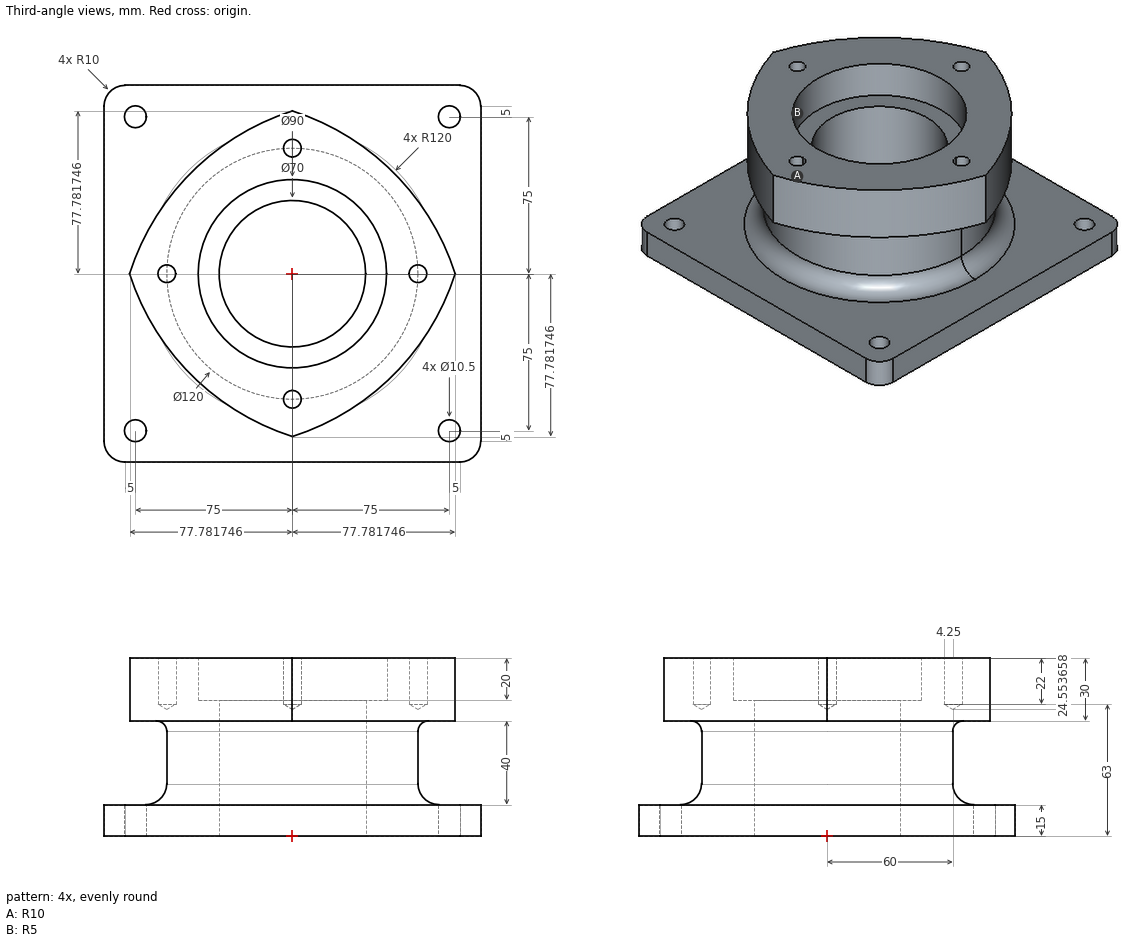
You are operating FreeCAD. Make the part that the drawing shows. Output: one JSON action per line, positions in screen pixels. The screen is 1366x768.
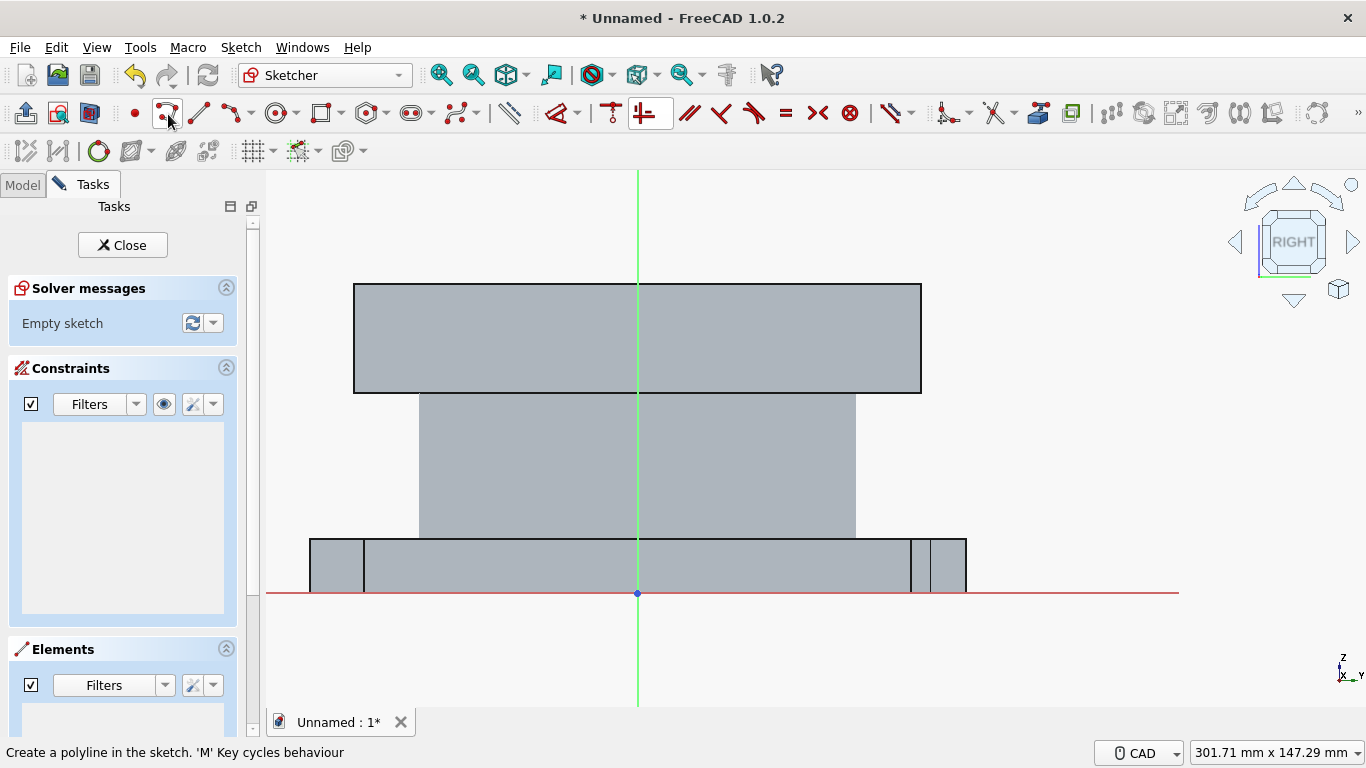
{"action": "left_click", "coordinate": [841, 364]}
{"action": "left_click", "coordinate": [857, 373]}
{"action": "left_click", "coordinate": [857, 284]}
{"action": "left_click", "coordinate": [841, 284]}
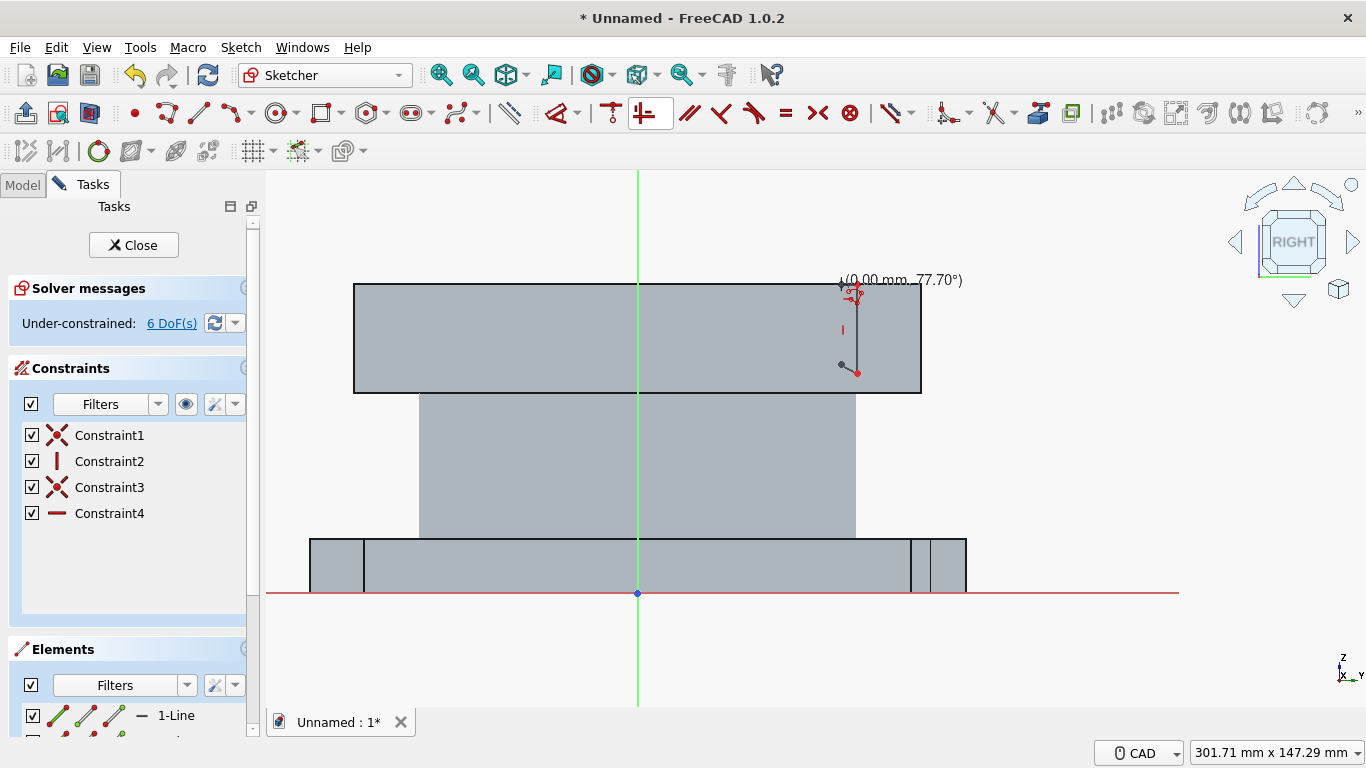
{"action": "scroll", "coordinate": [841, 364], "scroll_direction": "up", "scroll_amount": 3}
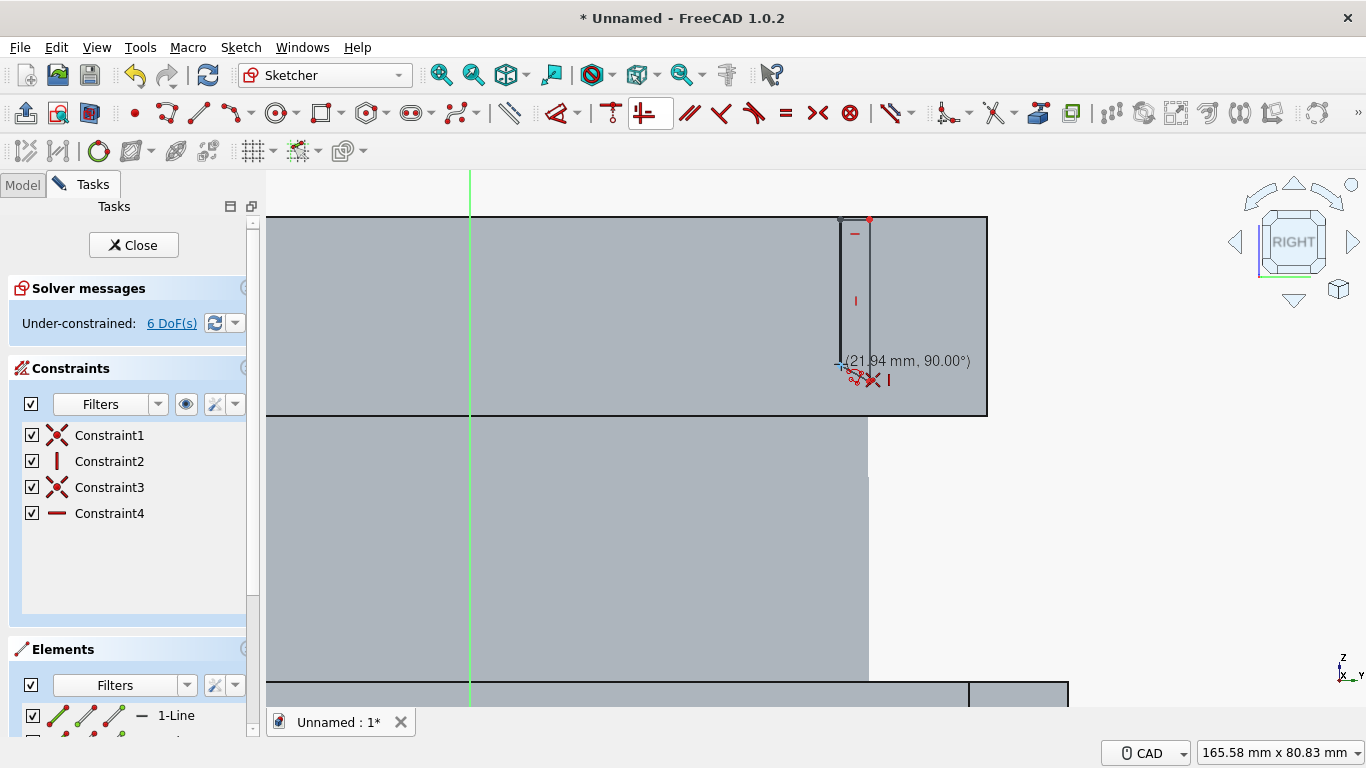
{"action": "left_click", "coordinate": [841, 366]}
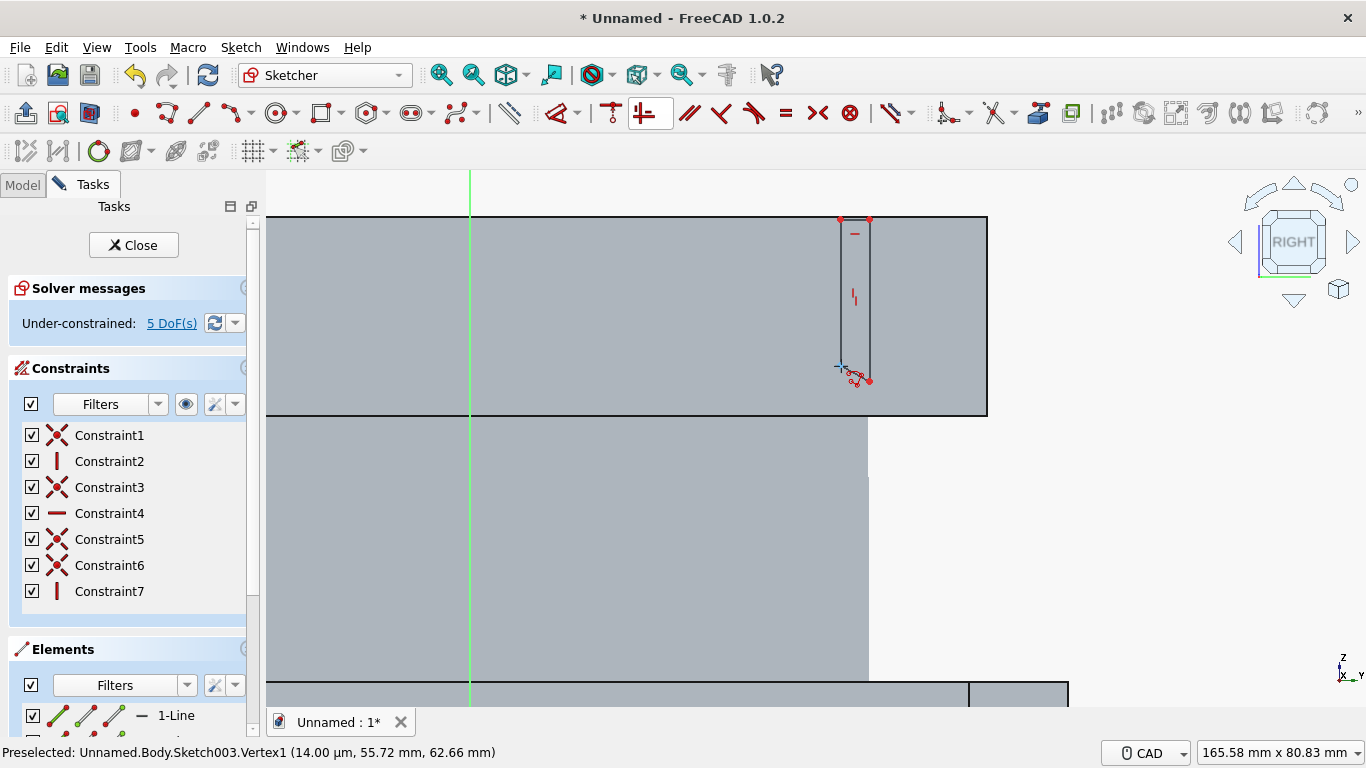
{"action": "left_click", "coordinate": [200, 114]}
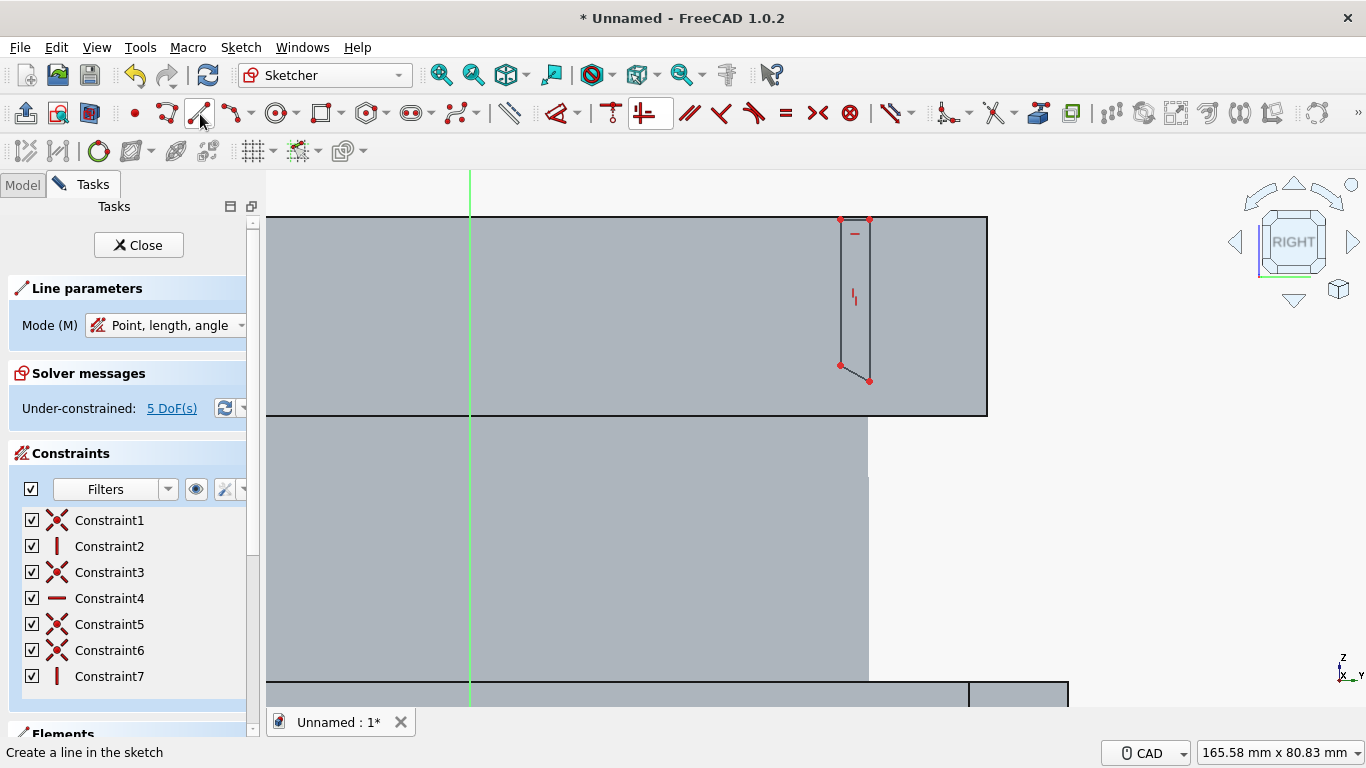
{"action": "left_click", "coordinate": [869, 397]}
{"action": "left_click", "coordinate": [869, 445]}
{"action": "key", "text": "Escape"}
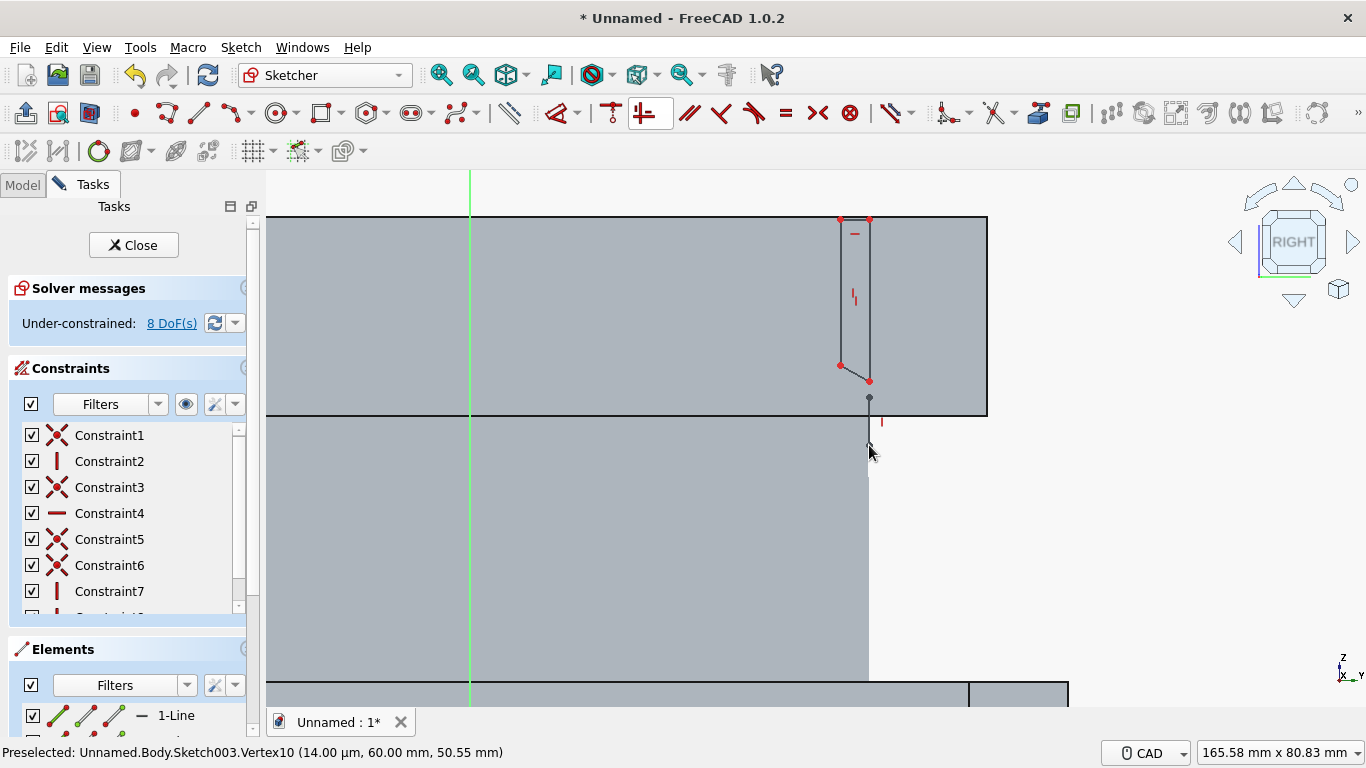
{"action": "left_click", "coordinate": [869, 412]}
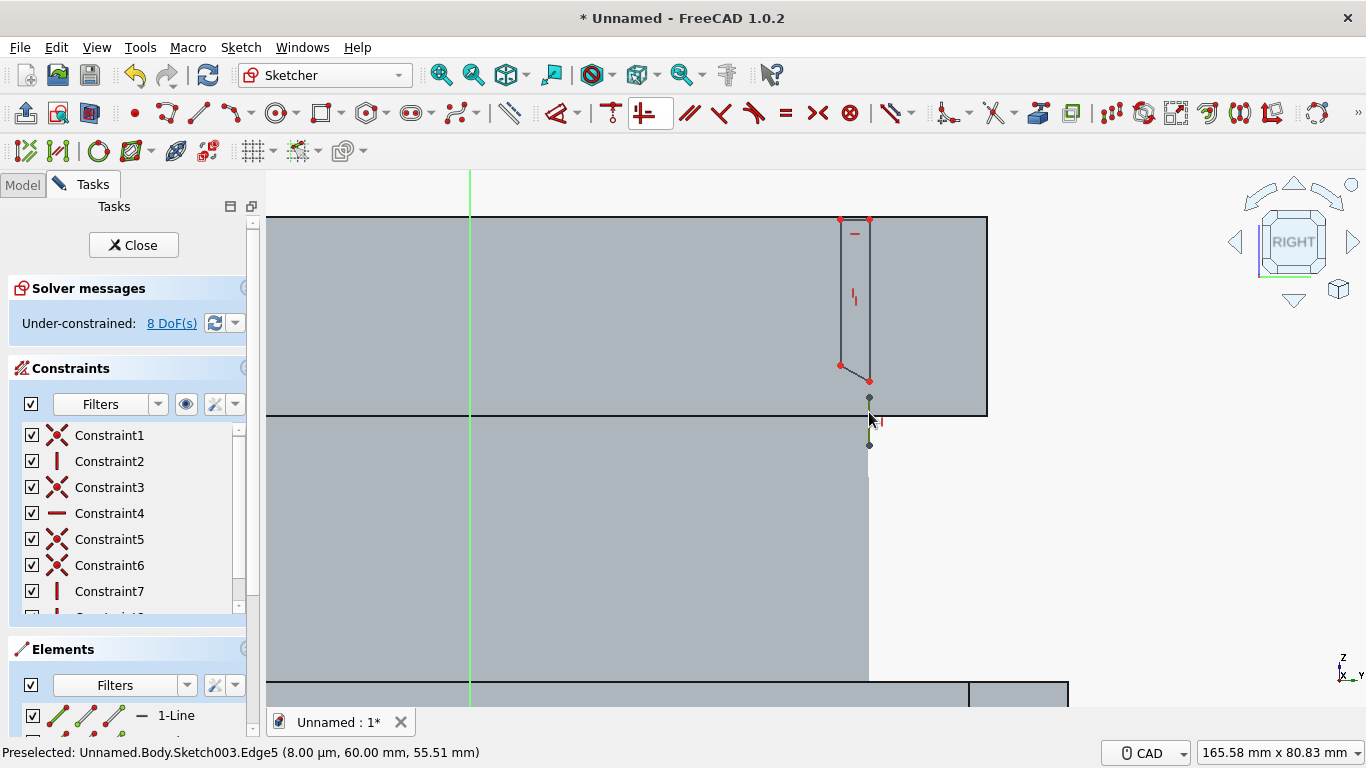
{"action": "left_click", "coordinate": [510, 114]}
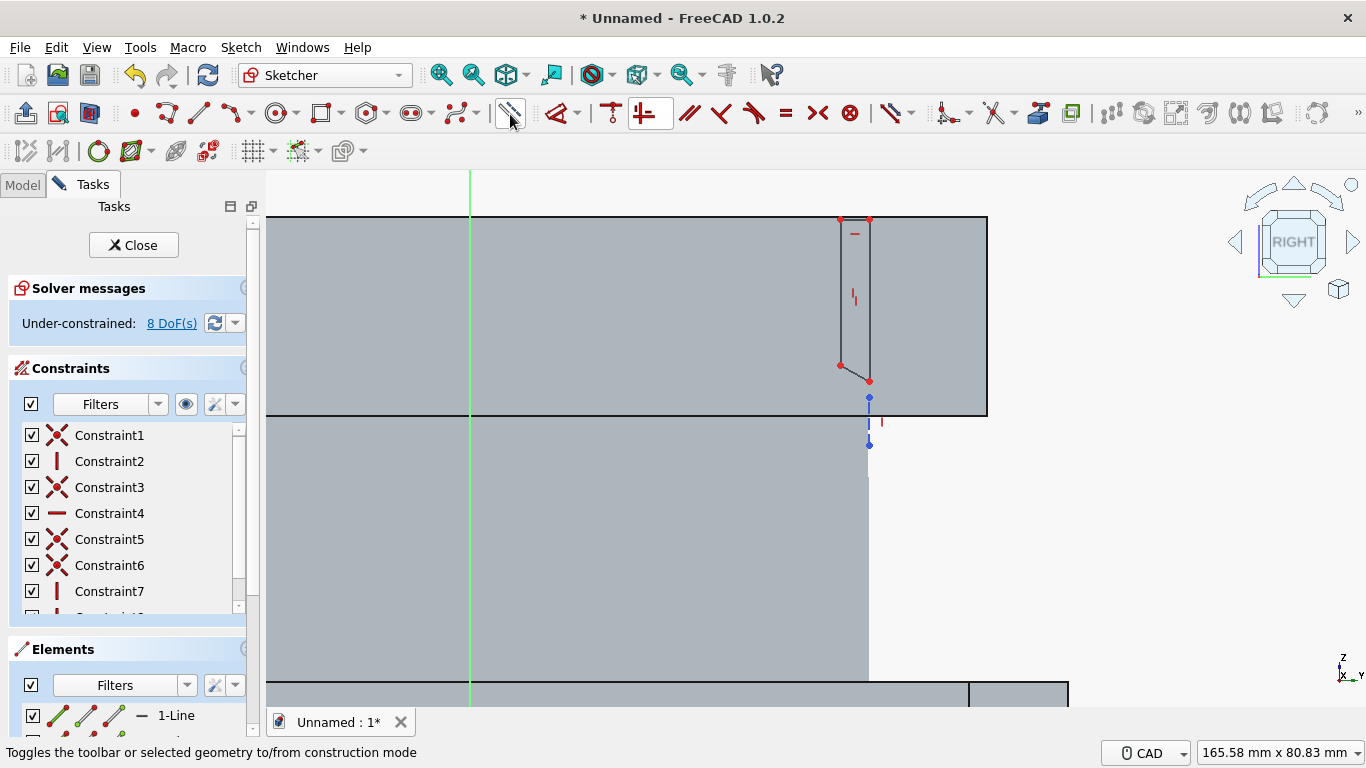
{"action": "left_click", "coordinate": [556, 114]}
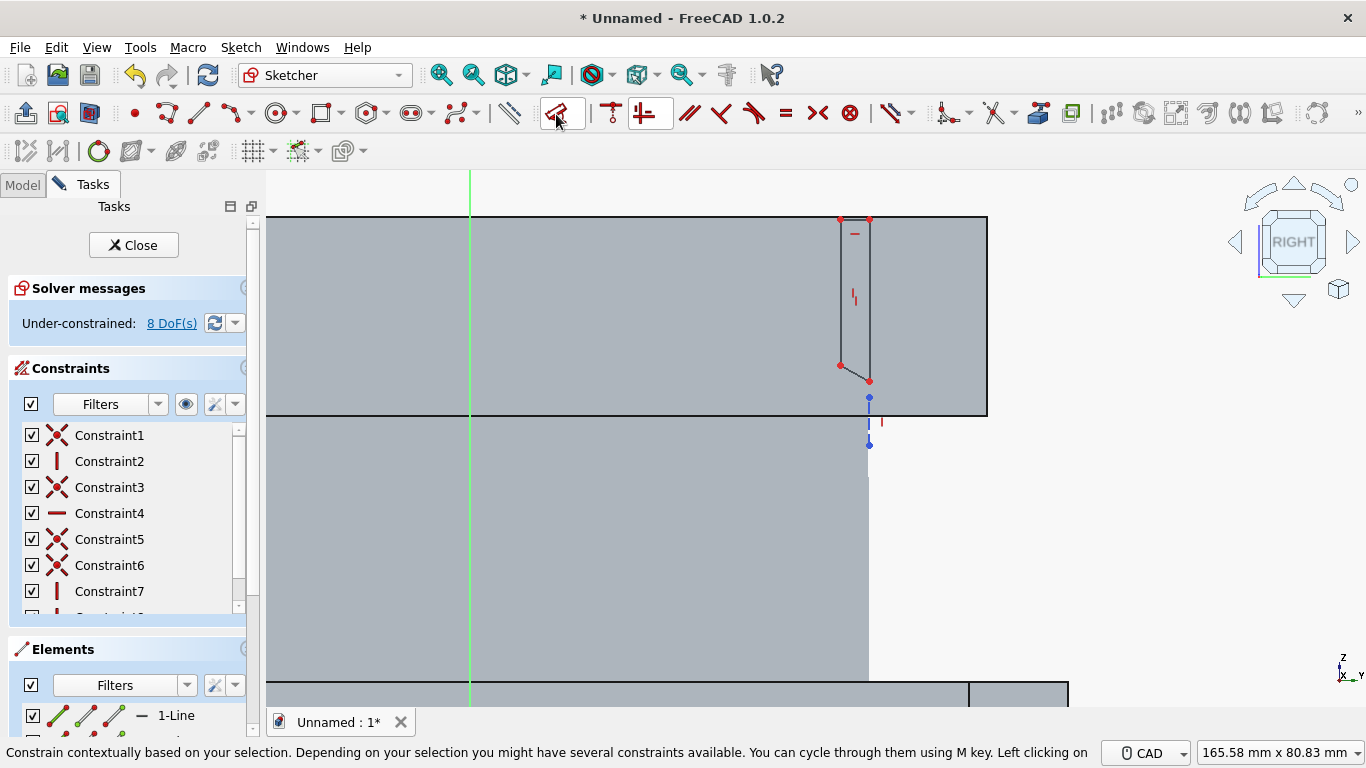
{"action": "left_click", "coordinate": [841, 263]}
{"action": "left_click", "coordinate": [807, 293]}